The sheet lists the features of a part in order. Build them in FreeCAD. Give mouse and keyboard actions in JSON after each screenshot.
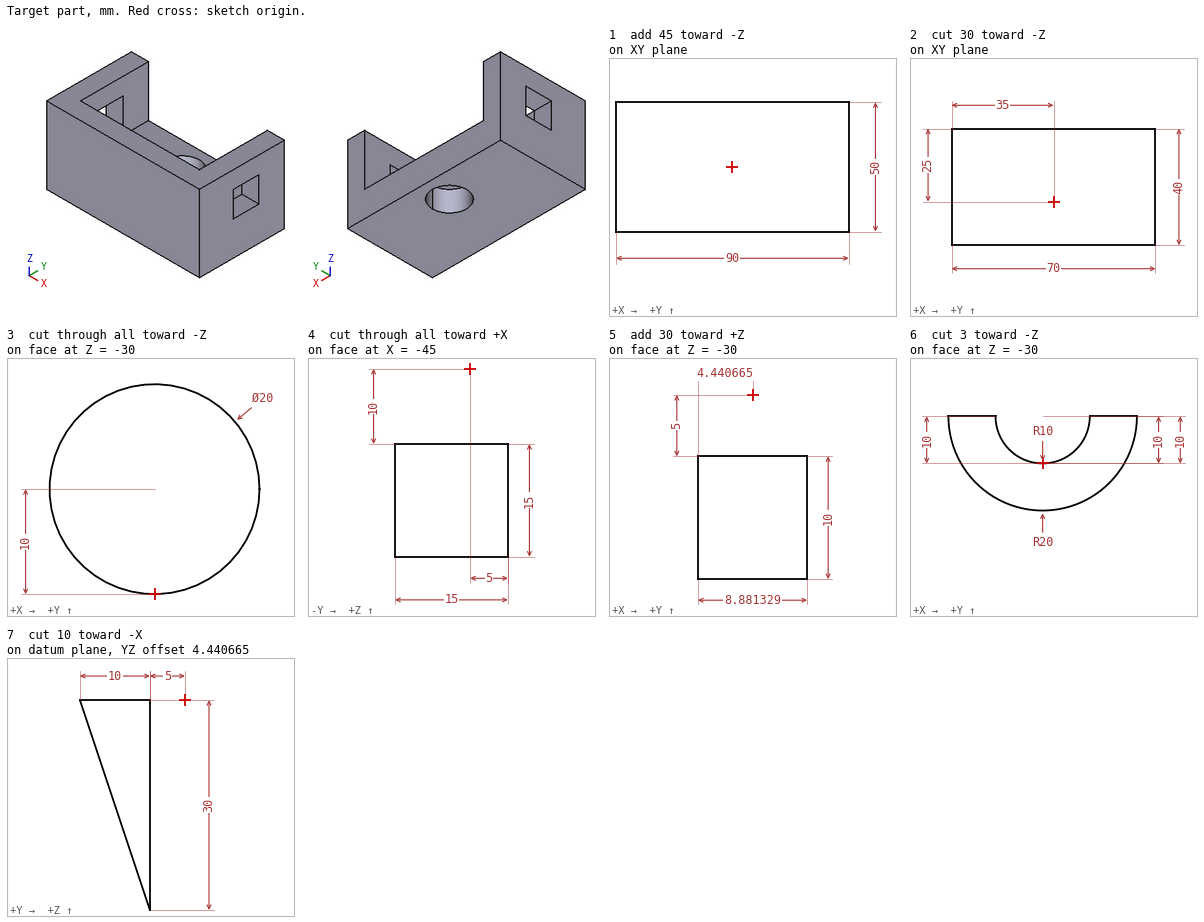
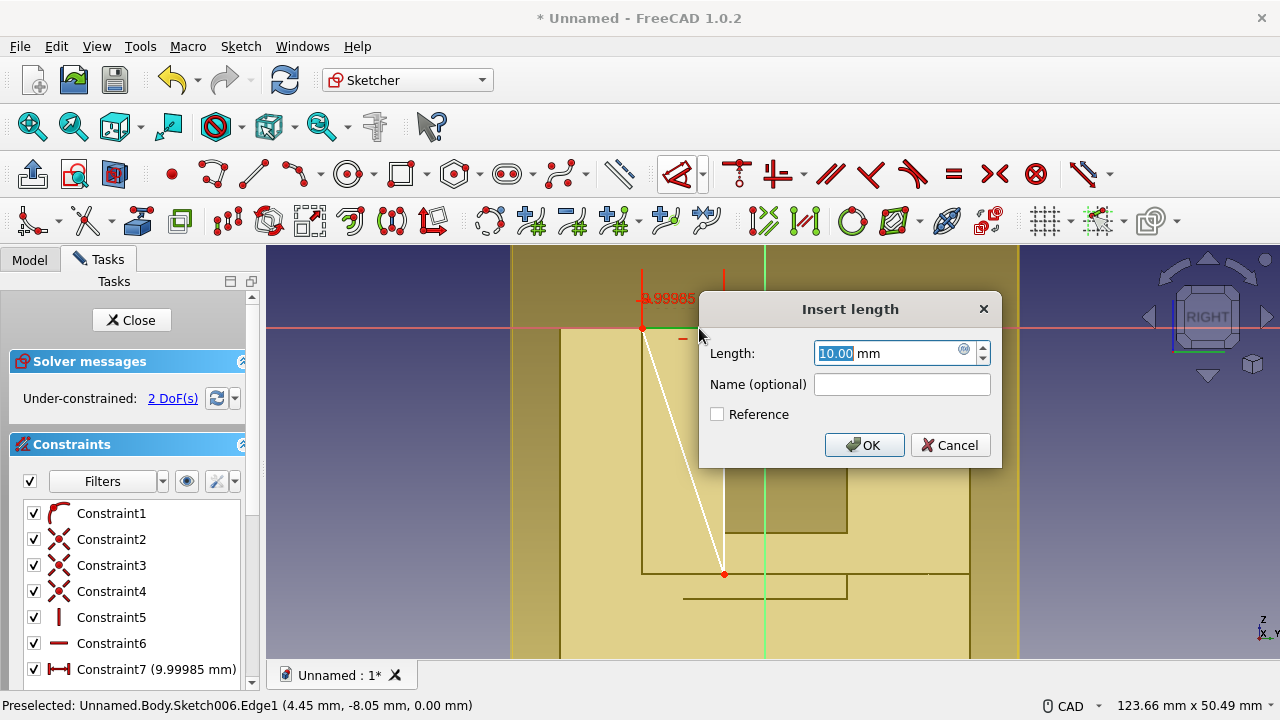
{"action": "type", "text": "10"}
{"action": "key", "text": "Return"}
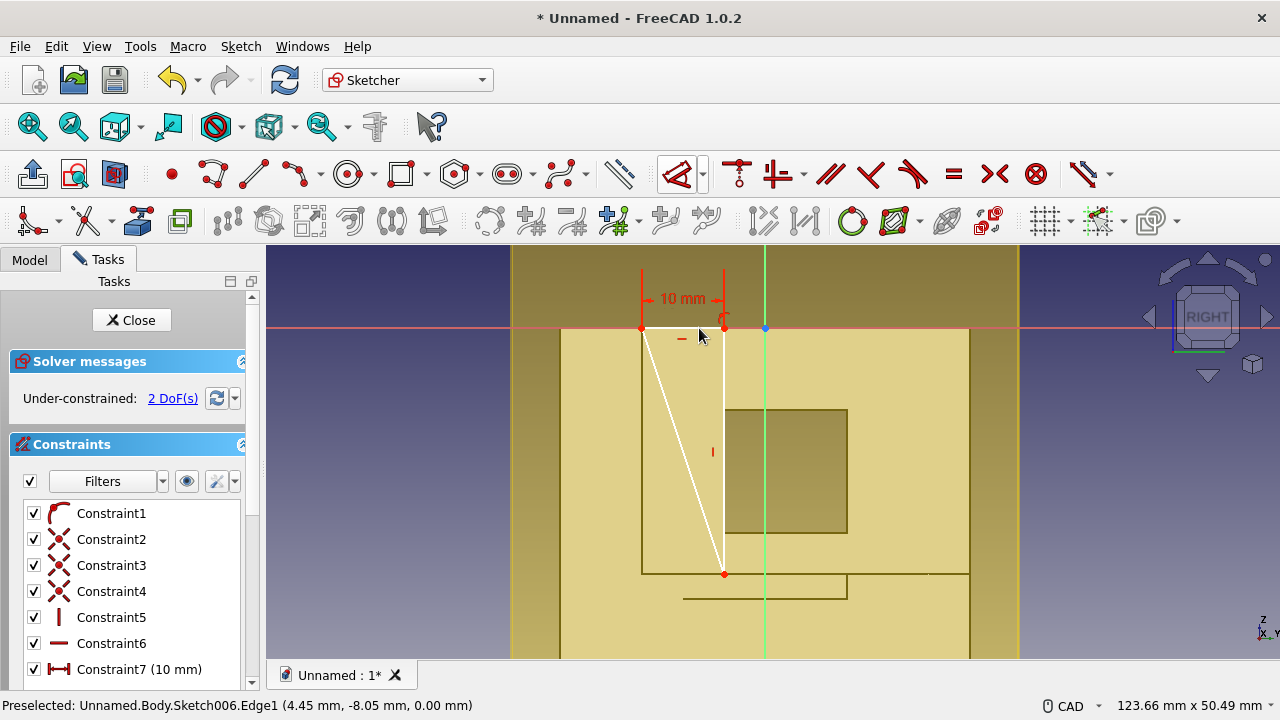
{"action": "left_click", "coordinate": [724, 501]}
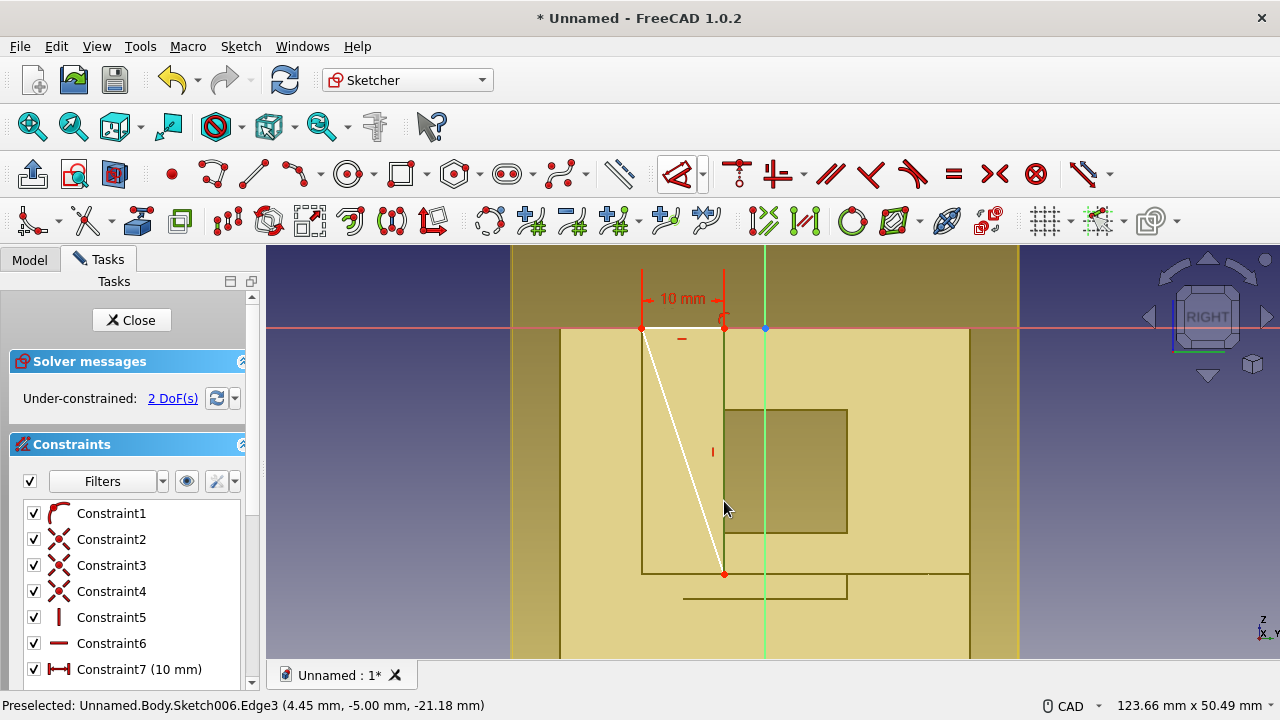
{"action": "key", "text": "i"}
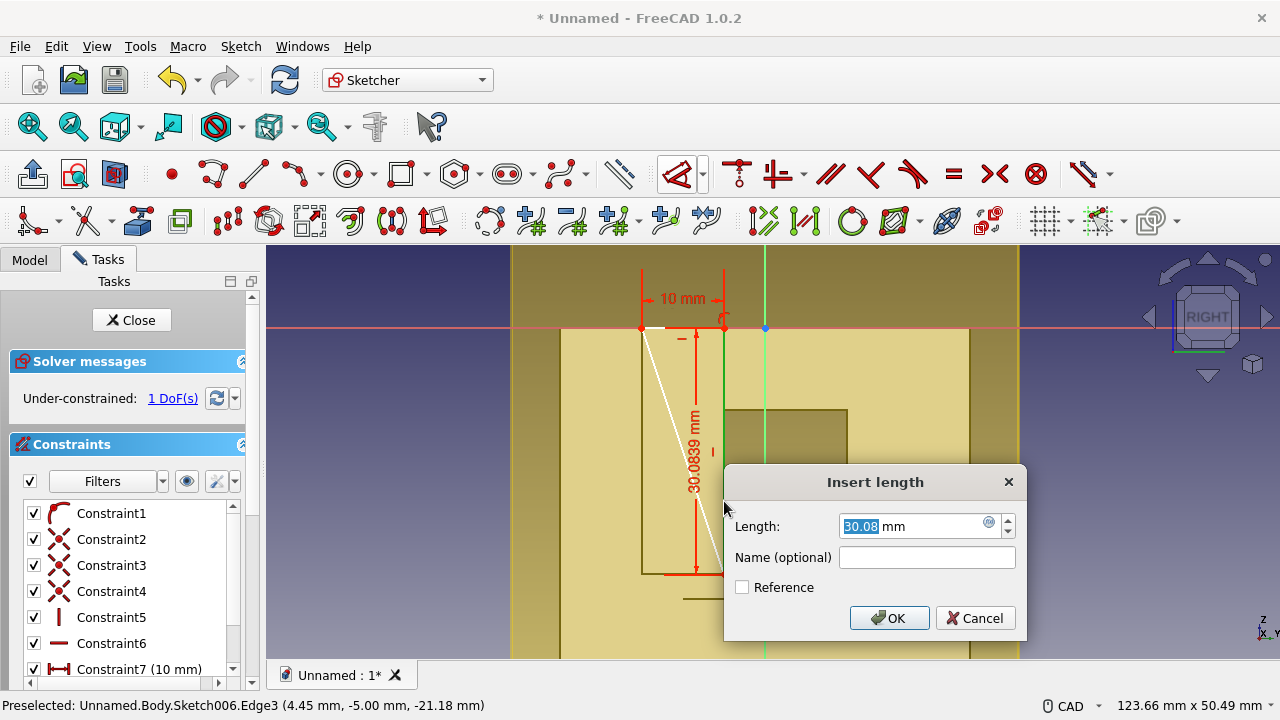
{"action": "type", "text": "30"}
{"action": "key", "text": "Return"}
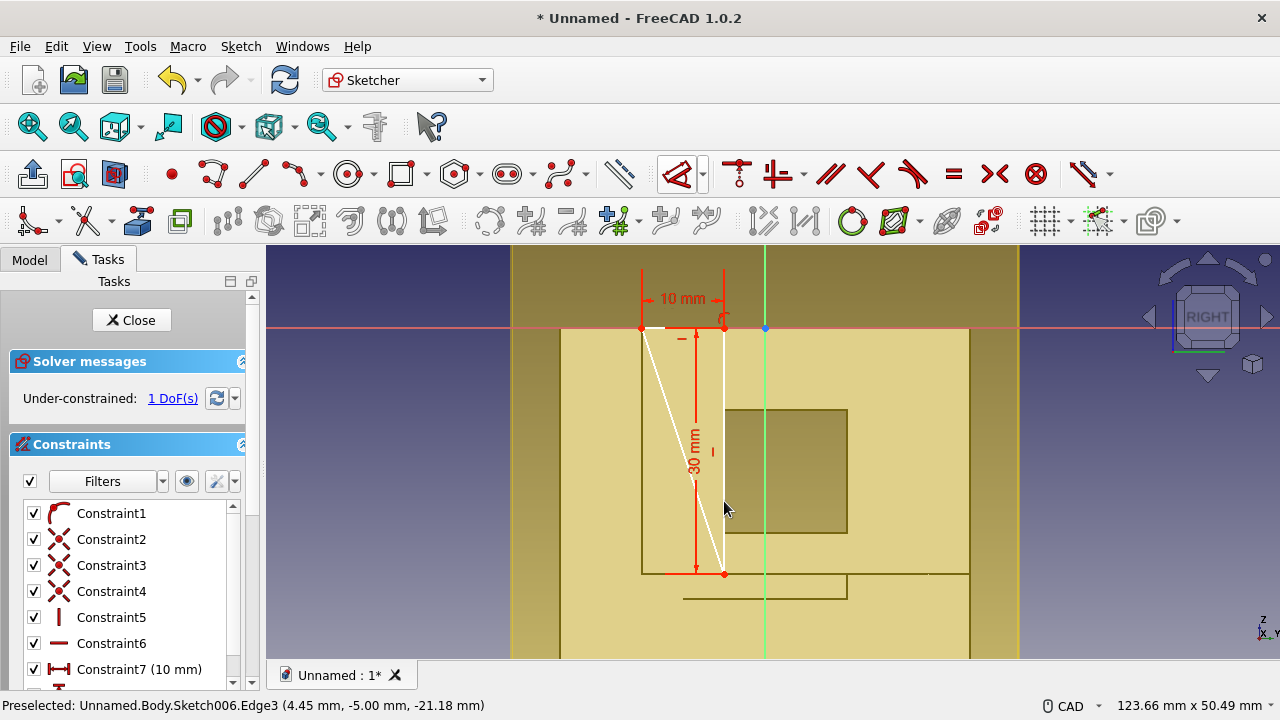
{"action": "left_click", "coordinate": [724, 328]}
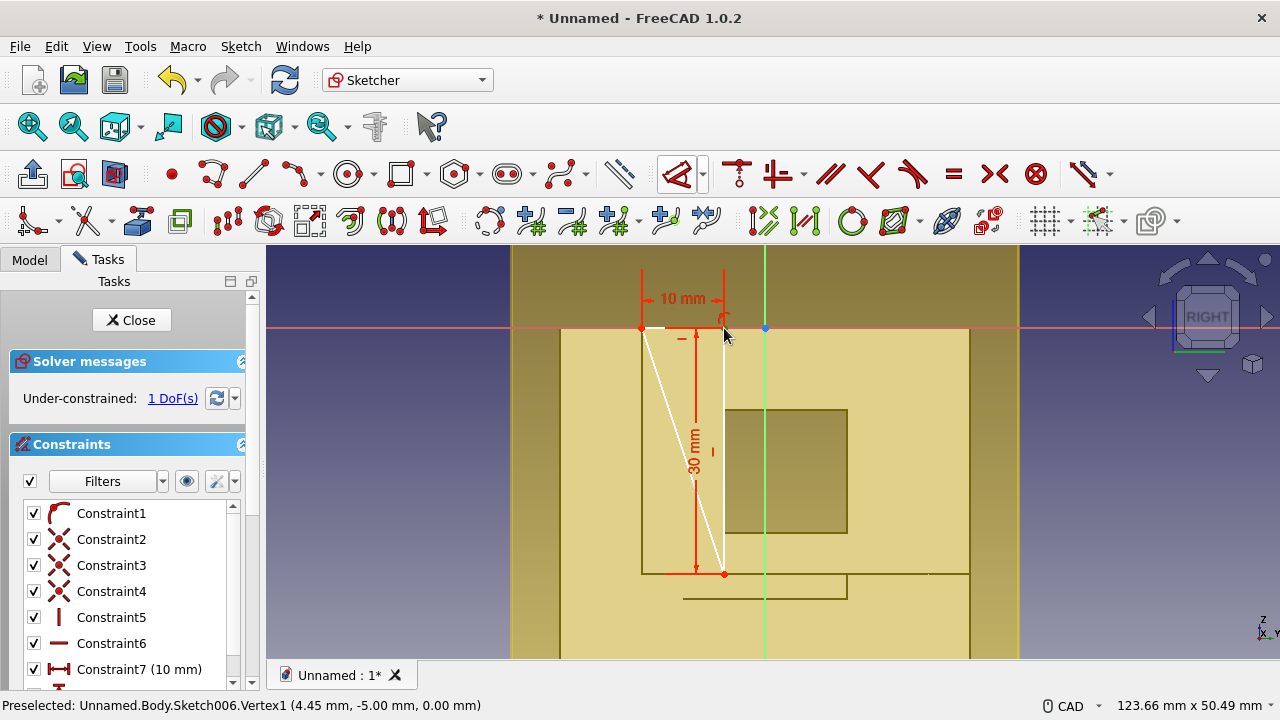
{"action": "key", "text": "l"}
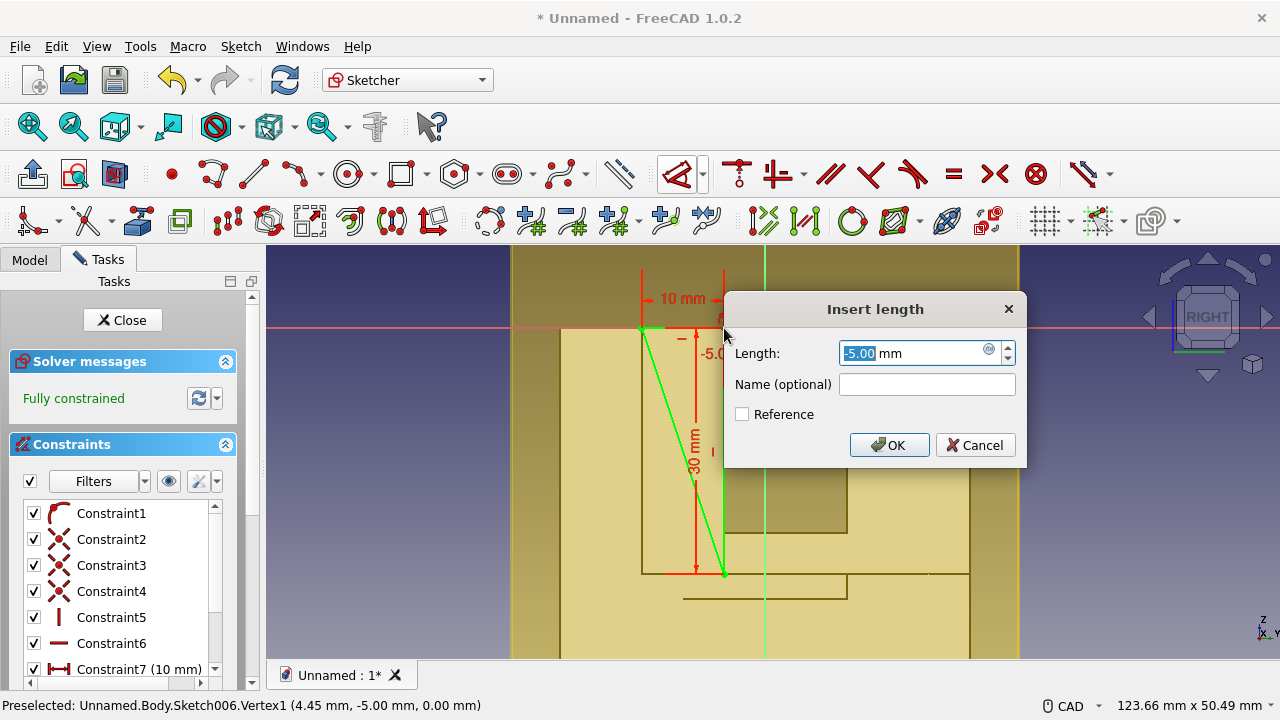
{"action": "type", "text": "-5"}
{"action": "key", "text": "Return"}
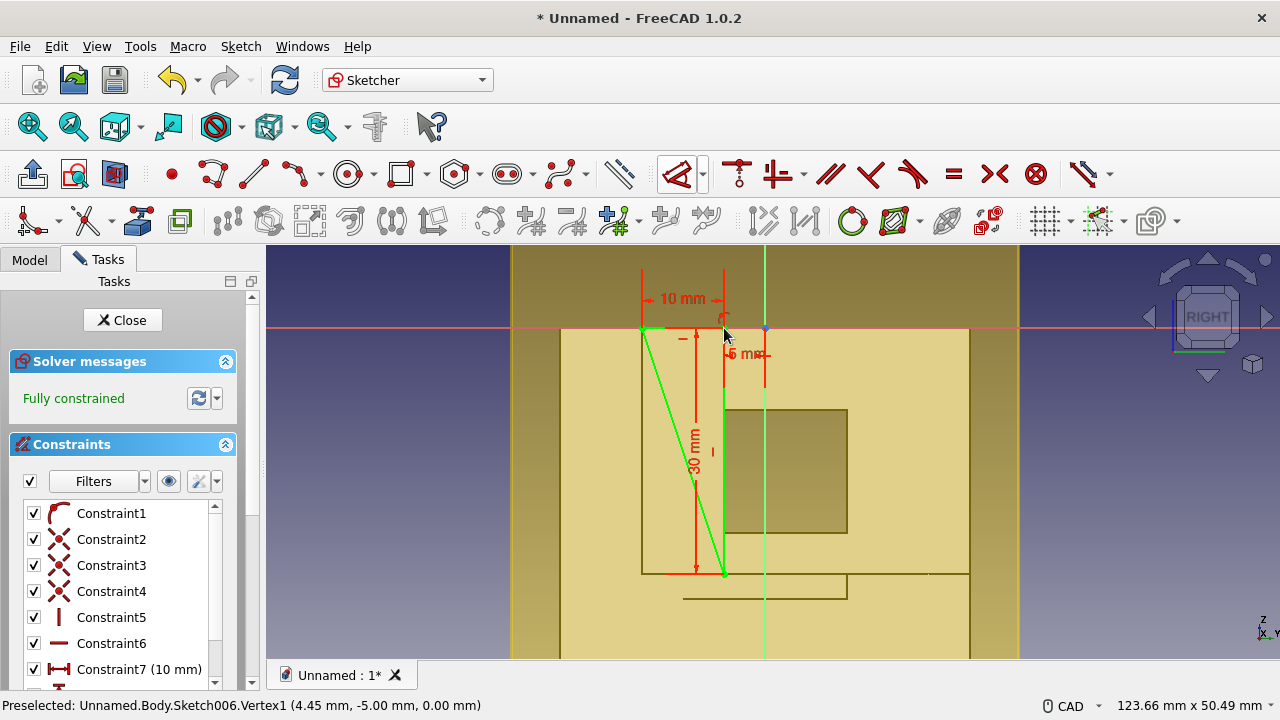
{"action": "left_click", "coordinate": [123, 320]}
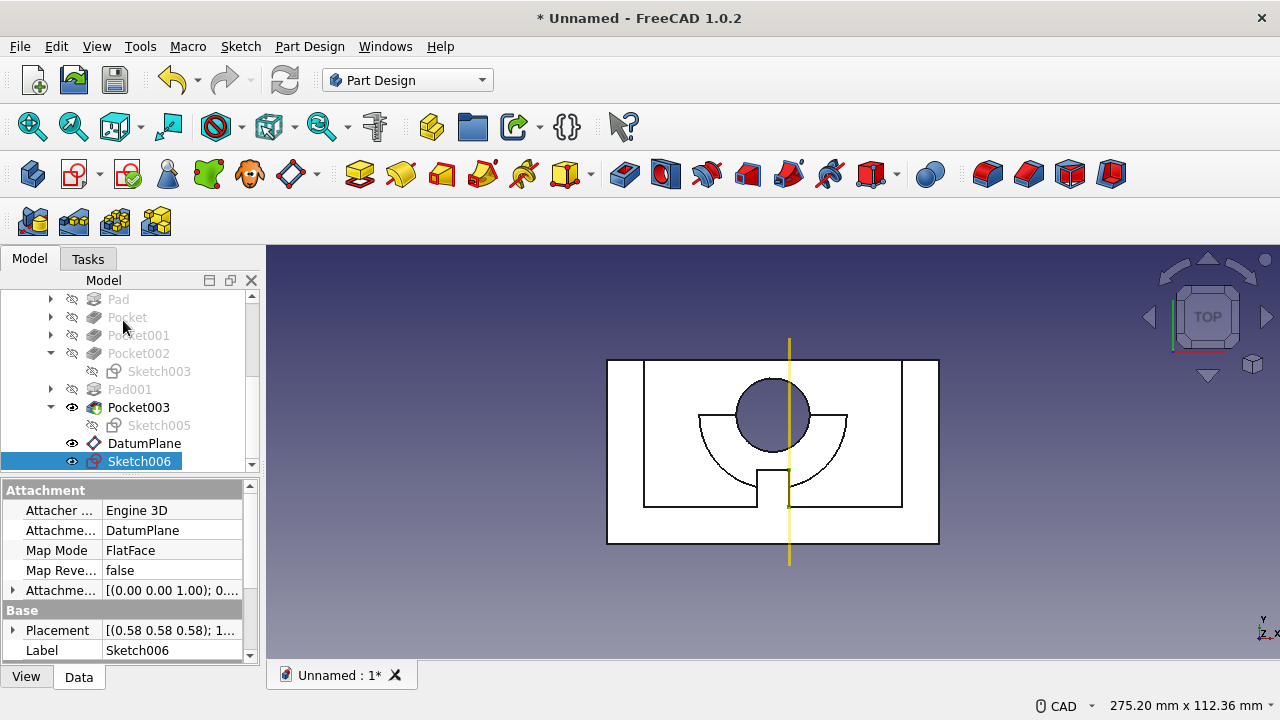
{"action": "left_click", "coordinate": [625, 174]}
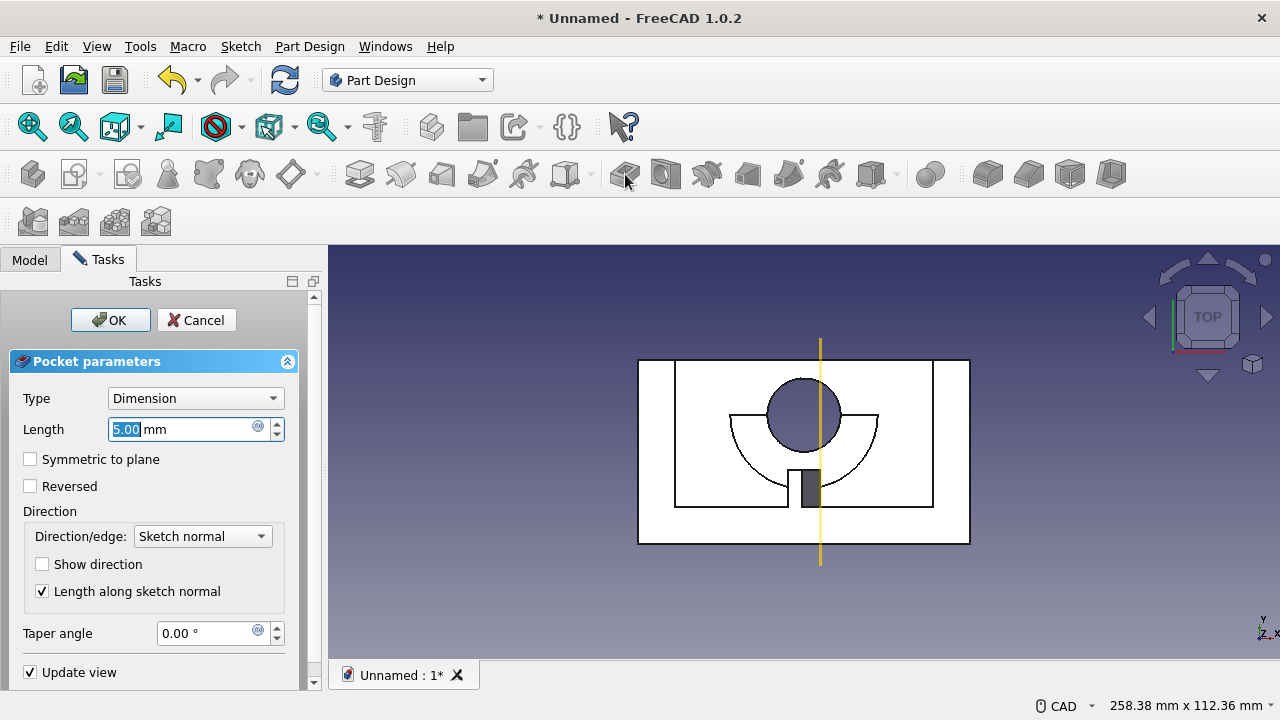
{"action": "type", "text": "10"}
{"action": "key", "text": "Tab"}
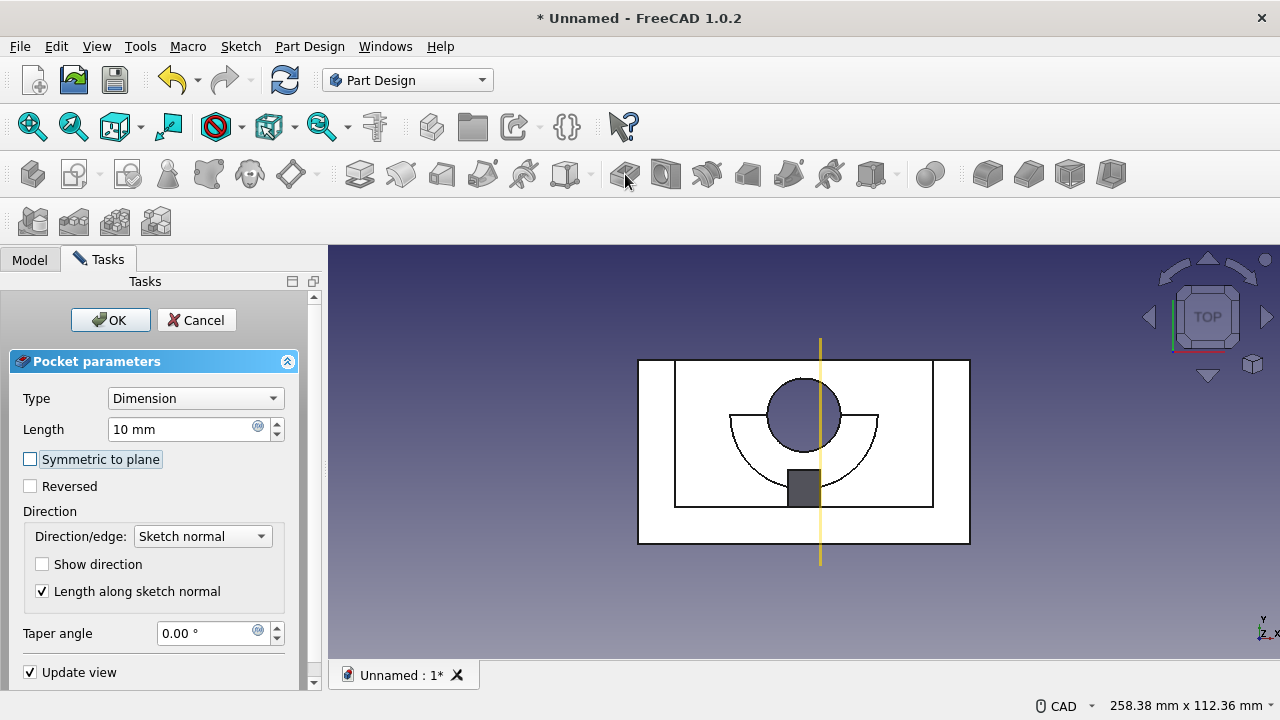
{"action": "left_click", "coordinate": [111, 320]}